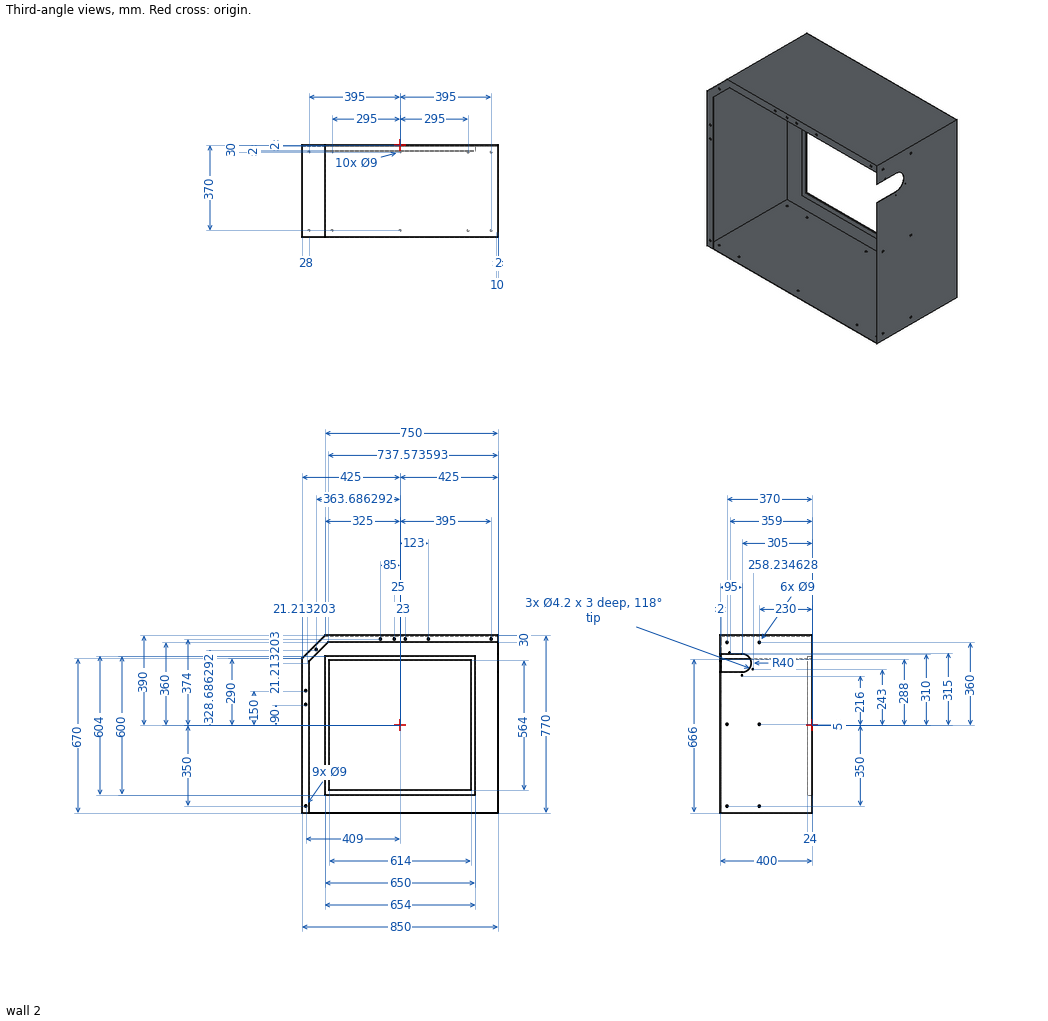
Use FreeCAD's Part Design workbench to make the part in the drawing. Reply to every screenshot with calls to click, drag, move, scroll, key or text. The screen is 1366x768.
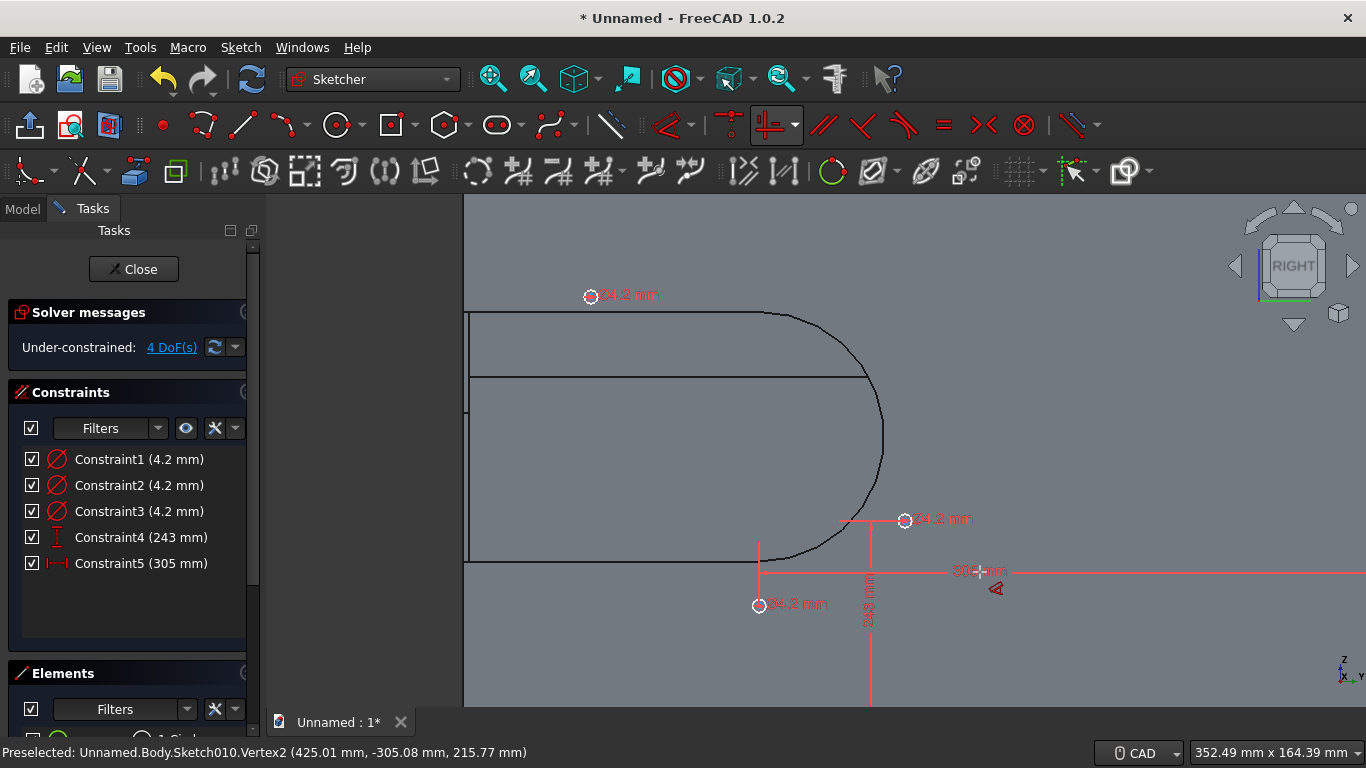
click(759, 606)
click(725, 642)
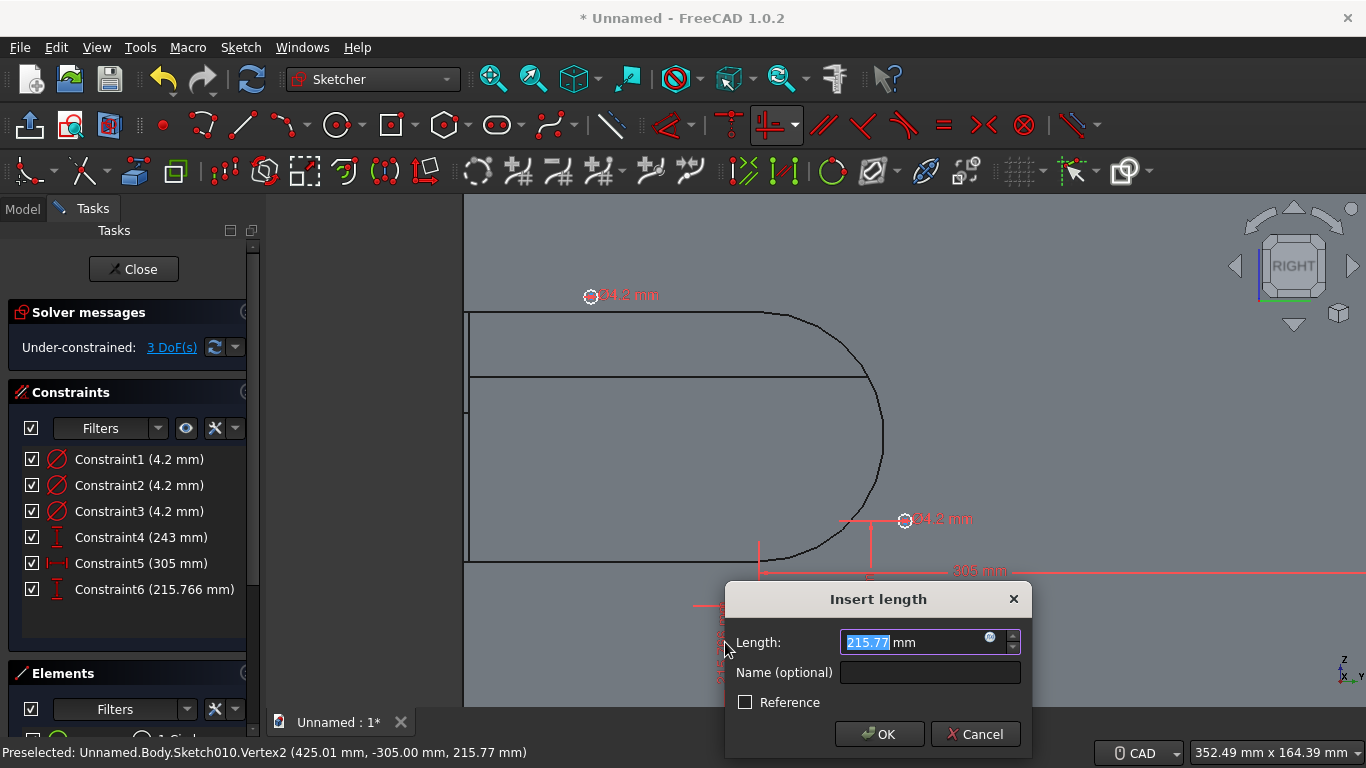
text(216)
key(Return)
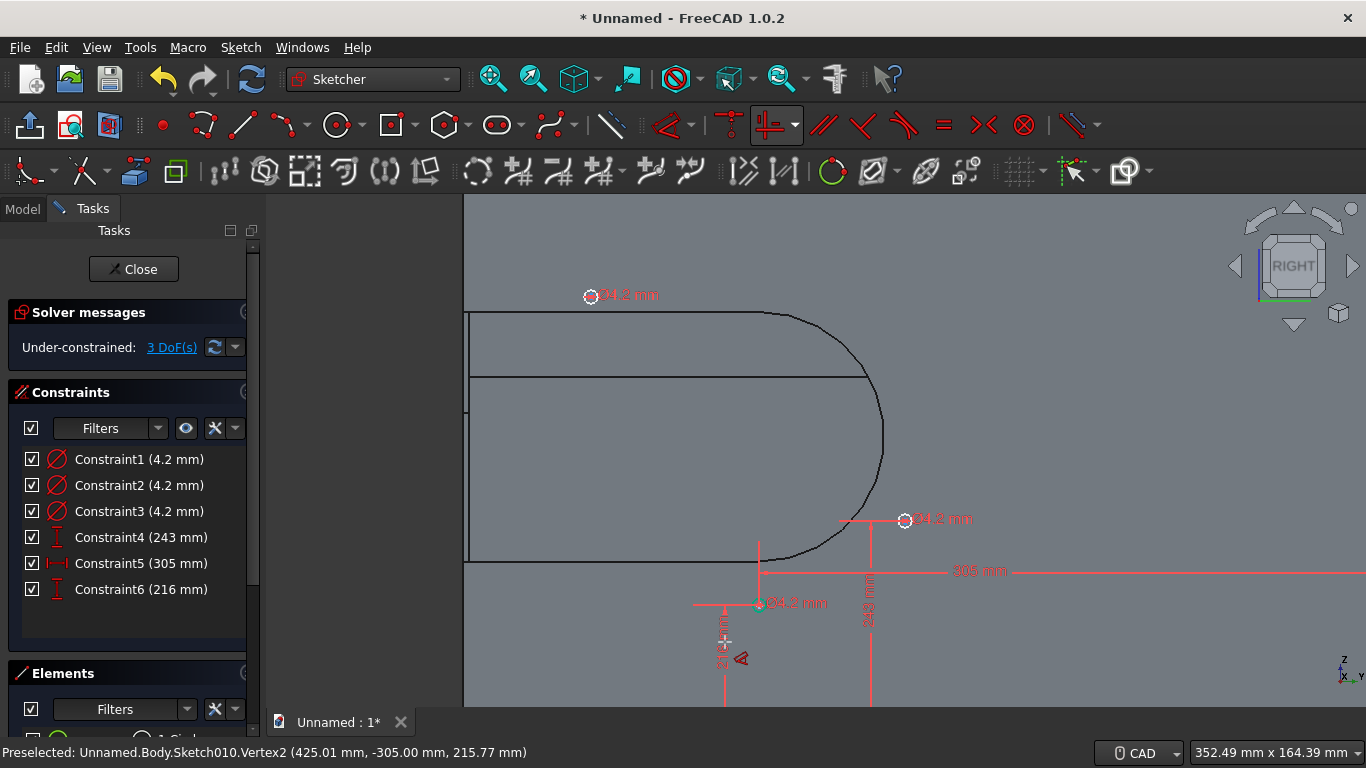
click(591, 297)
click(896, 263)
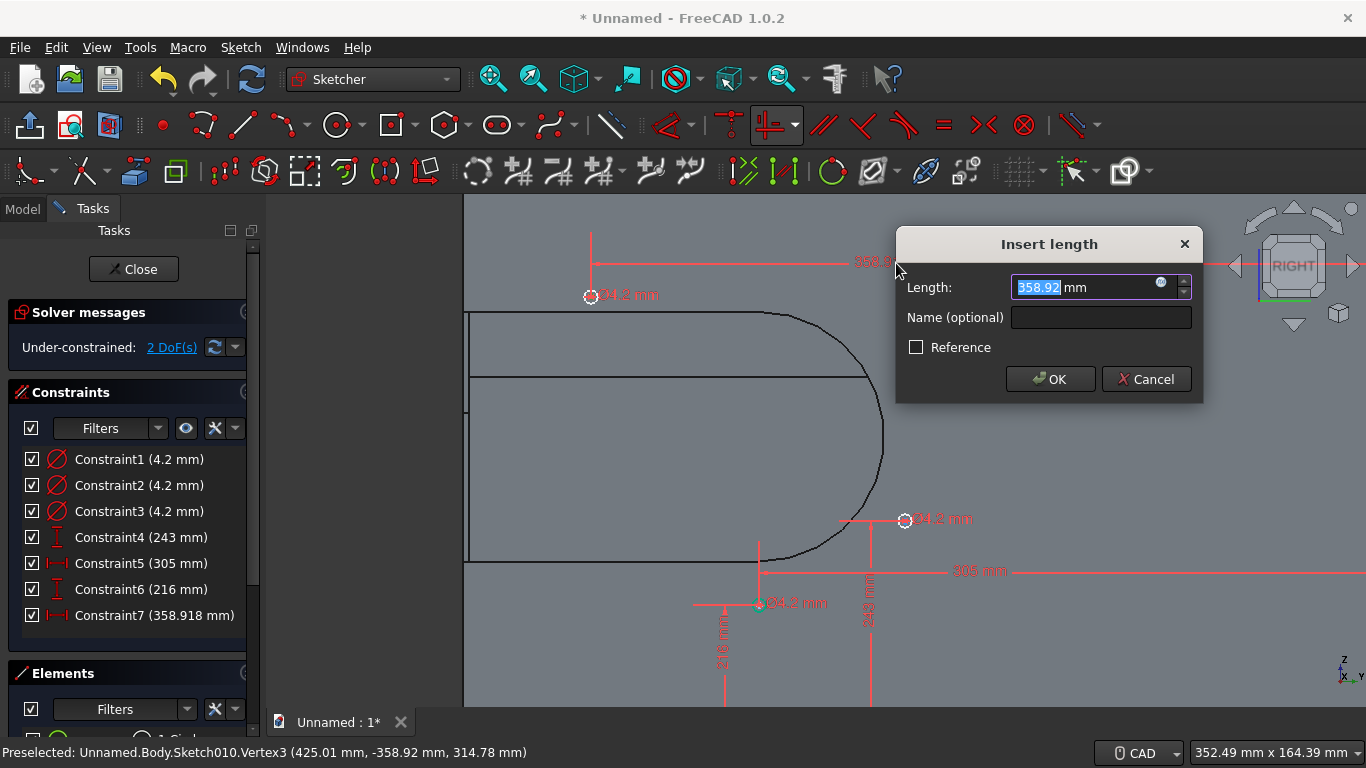
text(359)
key(Return)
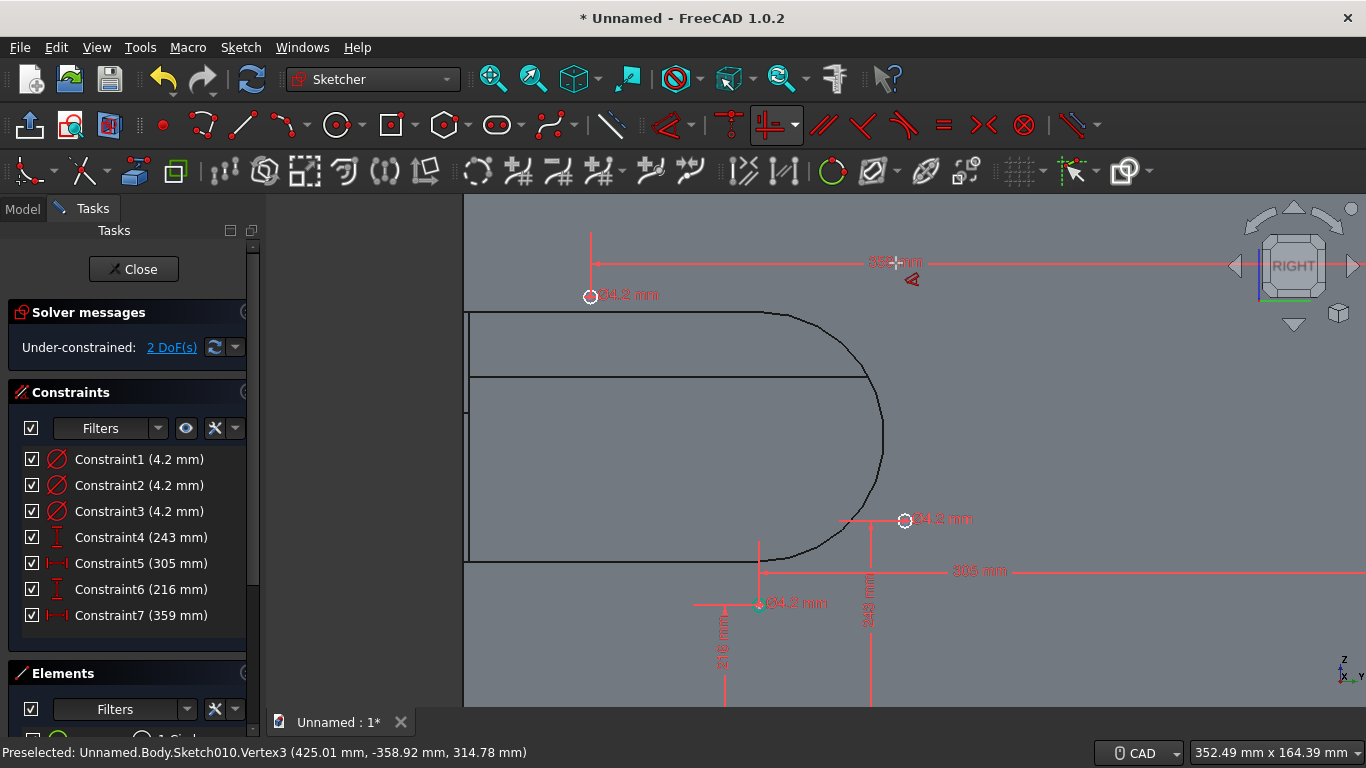
click(591, 297)
click(557, 488)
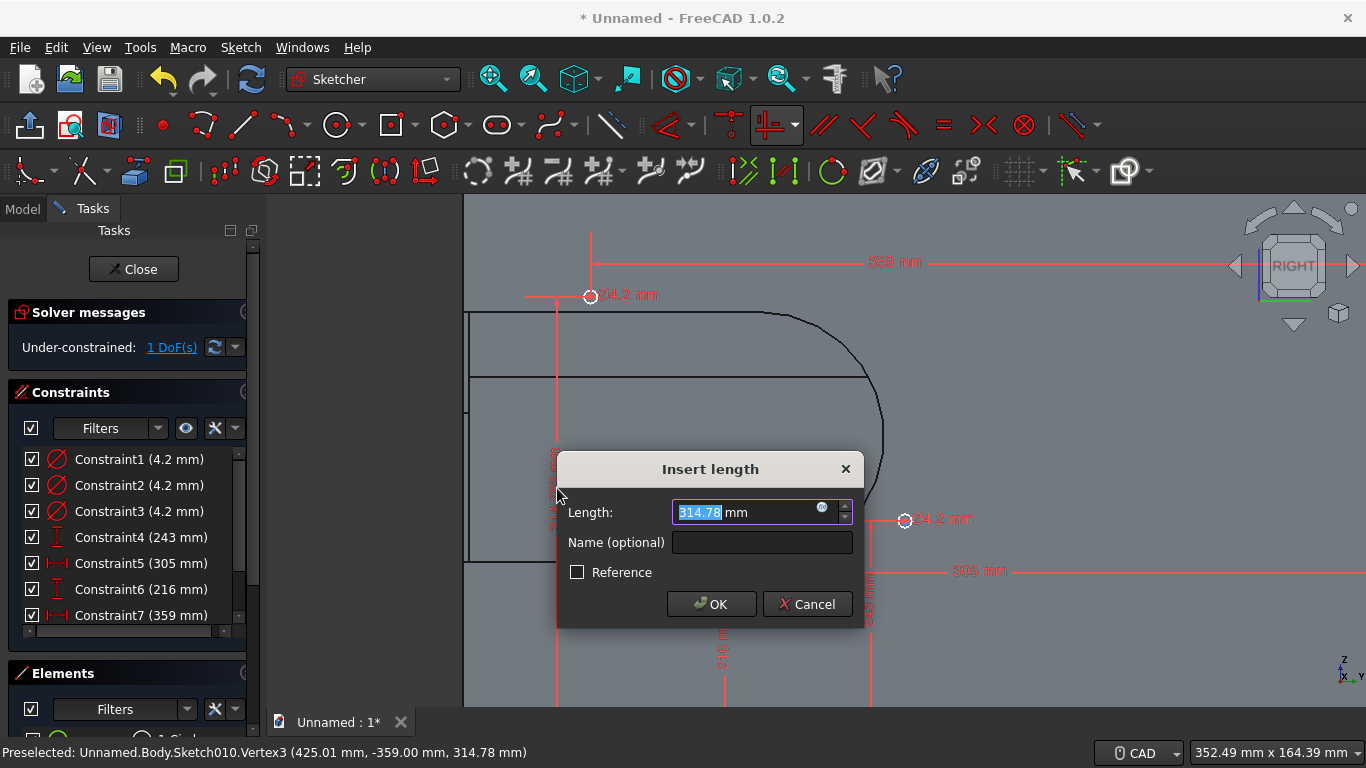
text(315)
key(Return)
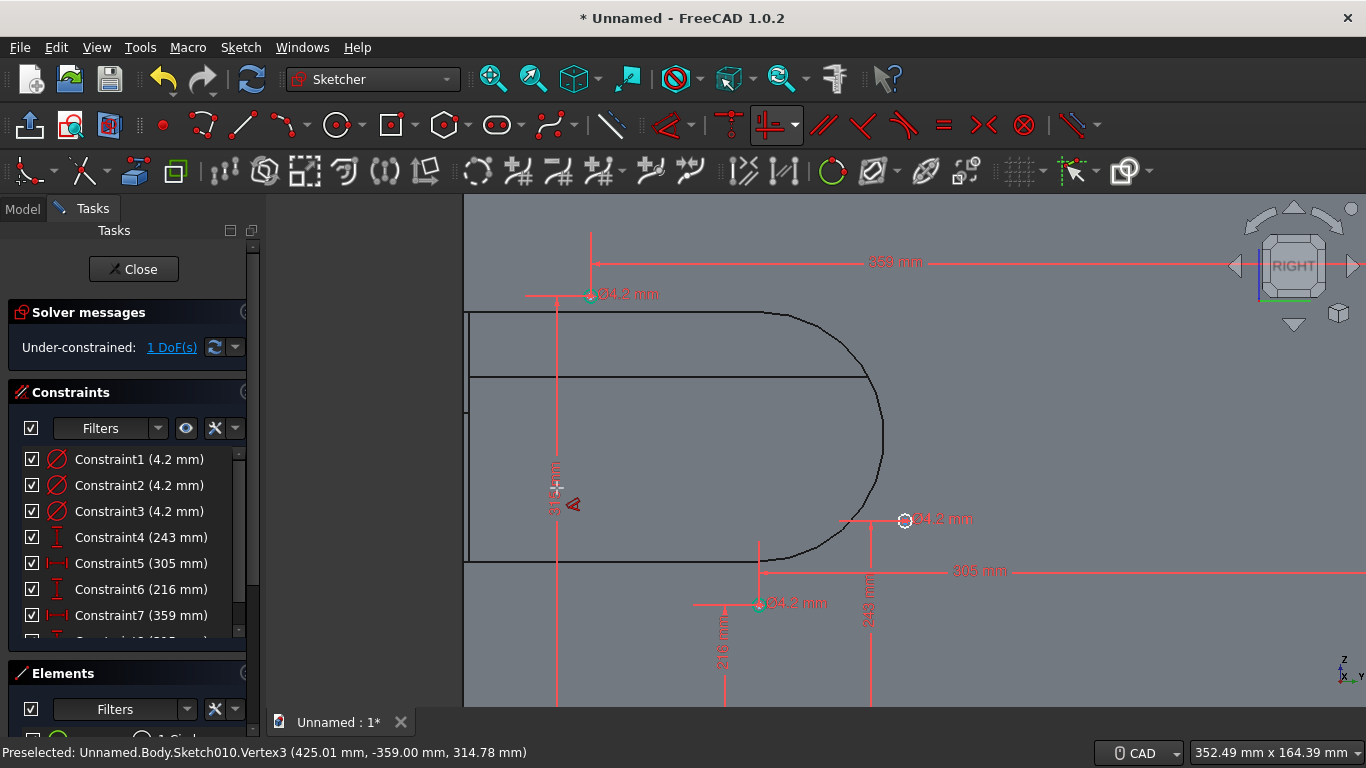
click(905, 521)
click(1053, 487)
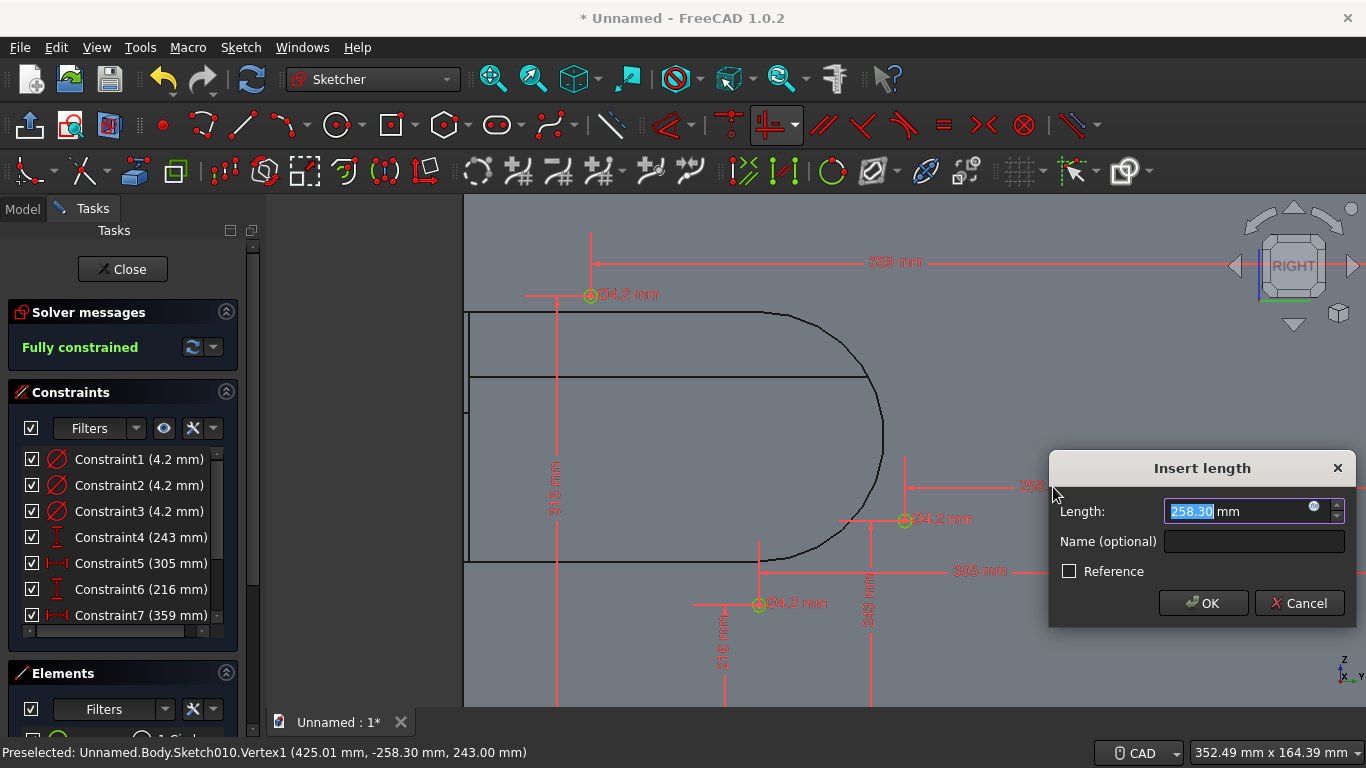
text(258.234628)
key(Return)
key(Escape)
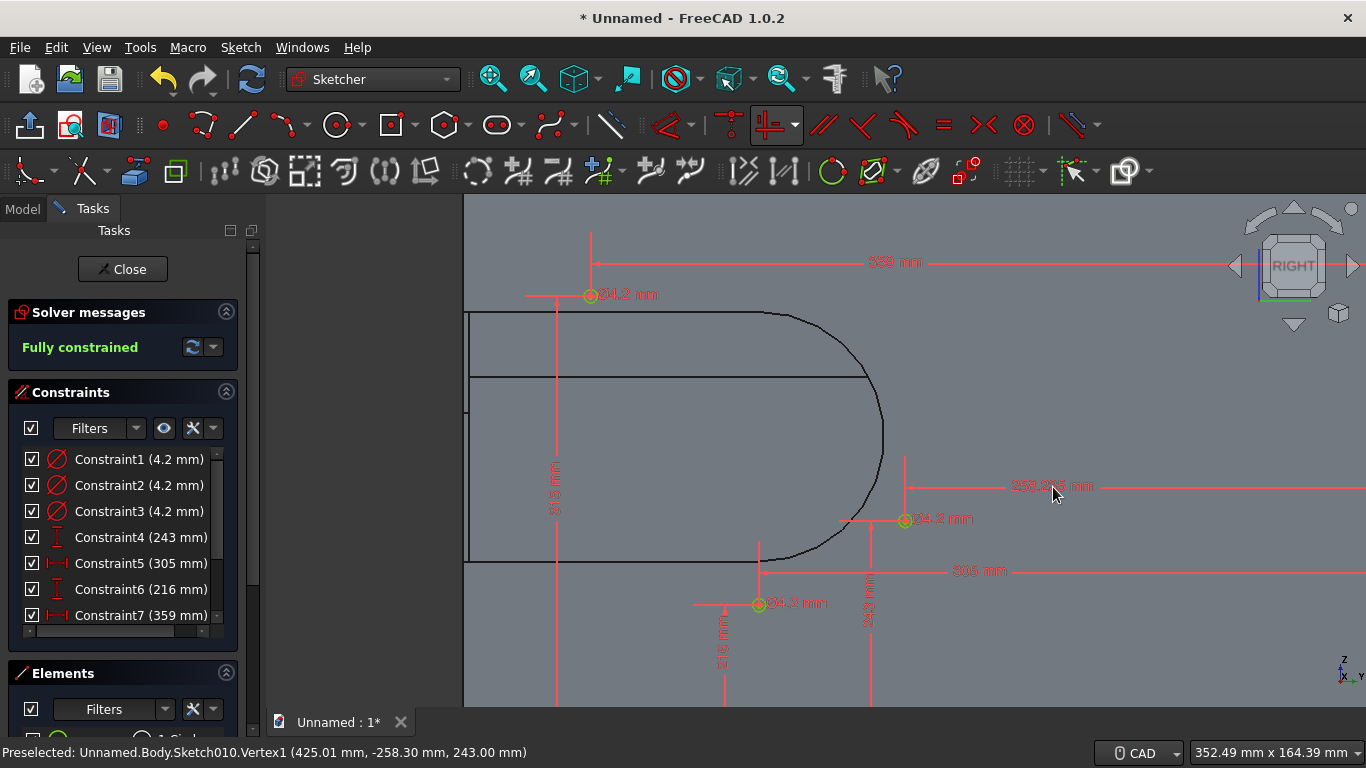
click(123, 269)